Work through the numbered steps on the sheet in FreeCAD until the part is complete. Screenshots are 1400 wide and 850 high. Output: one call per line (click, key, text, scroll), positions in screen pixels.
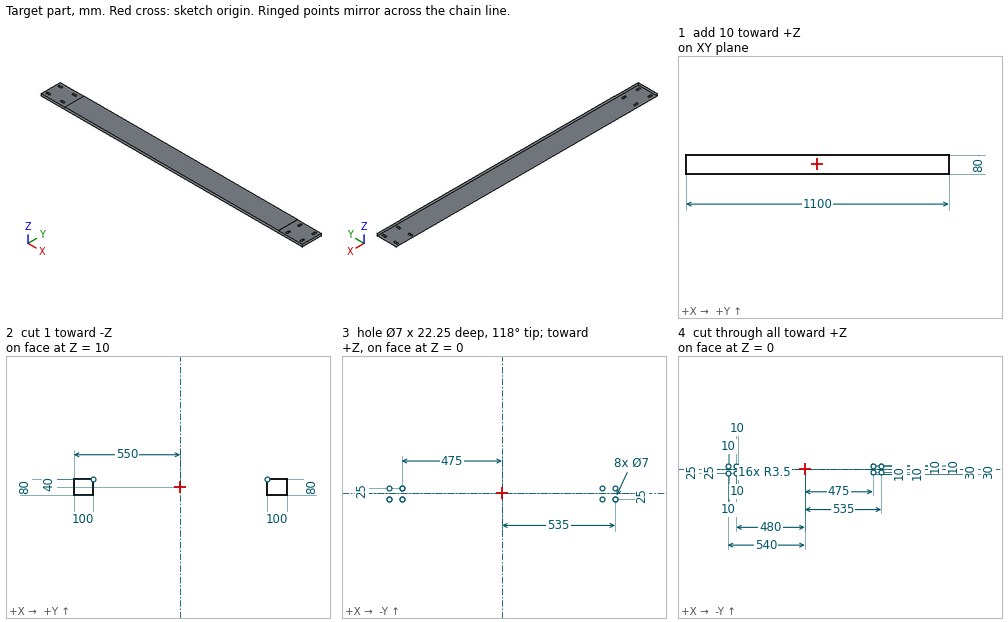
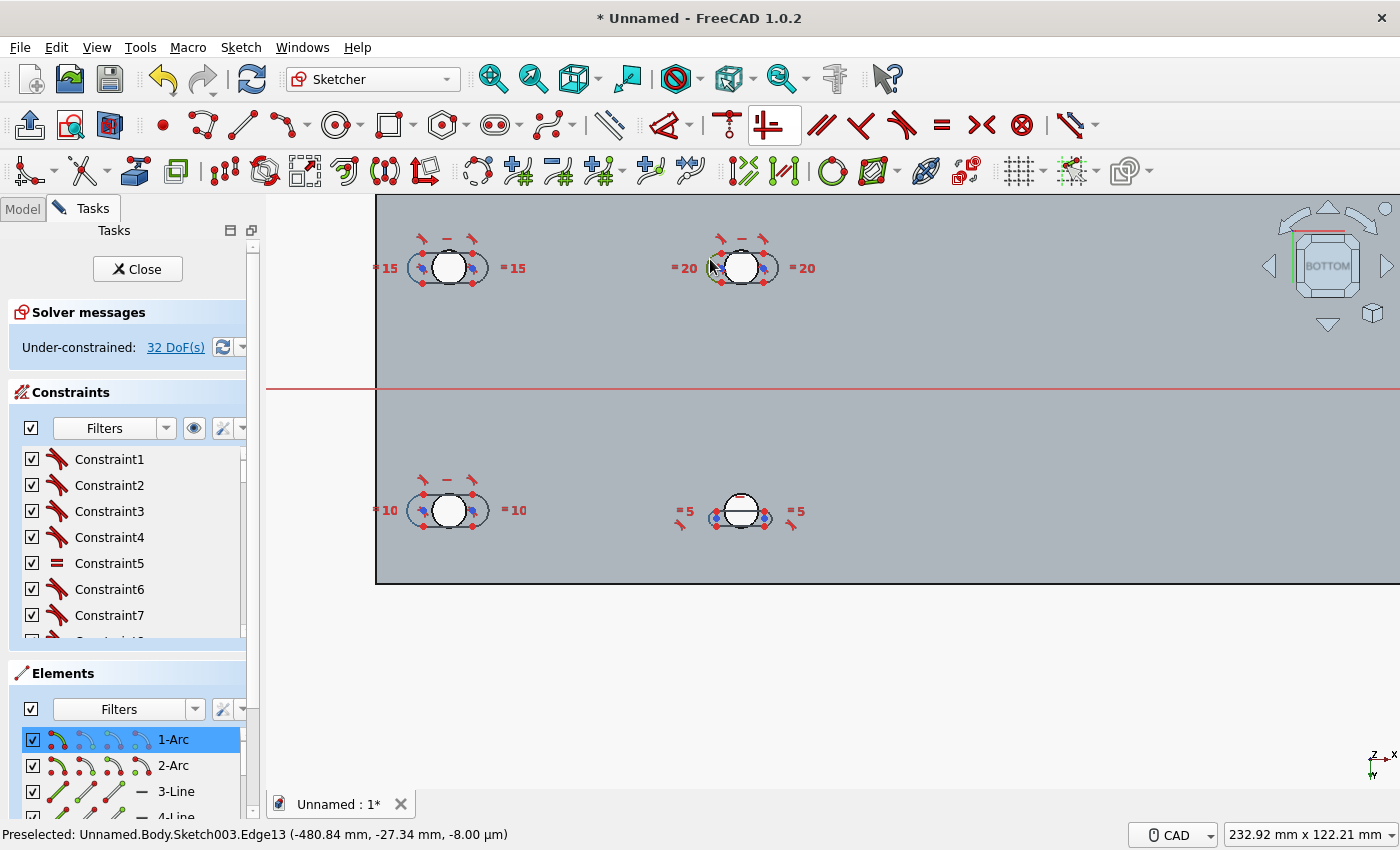
scroll(408, 508, down, 10)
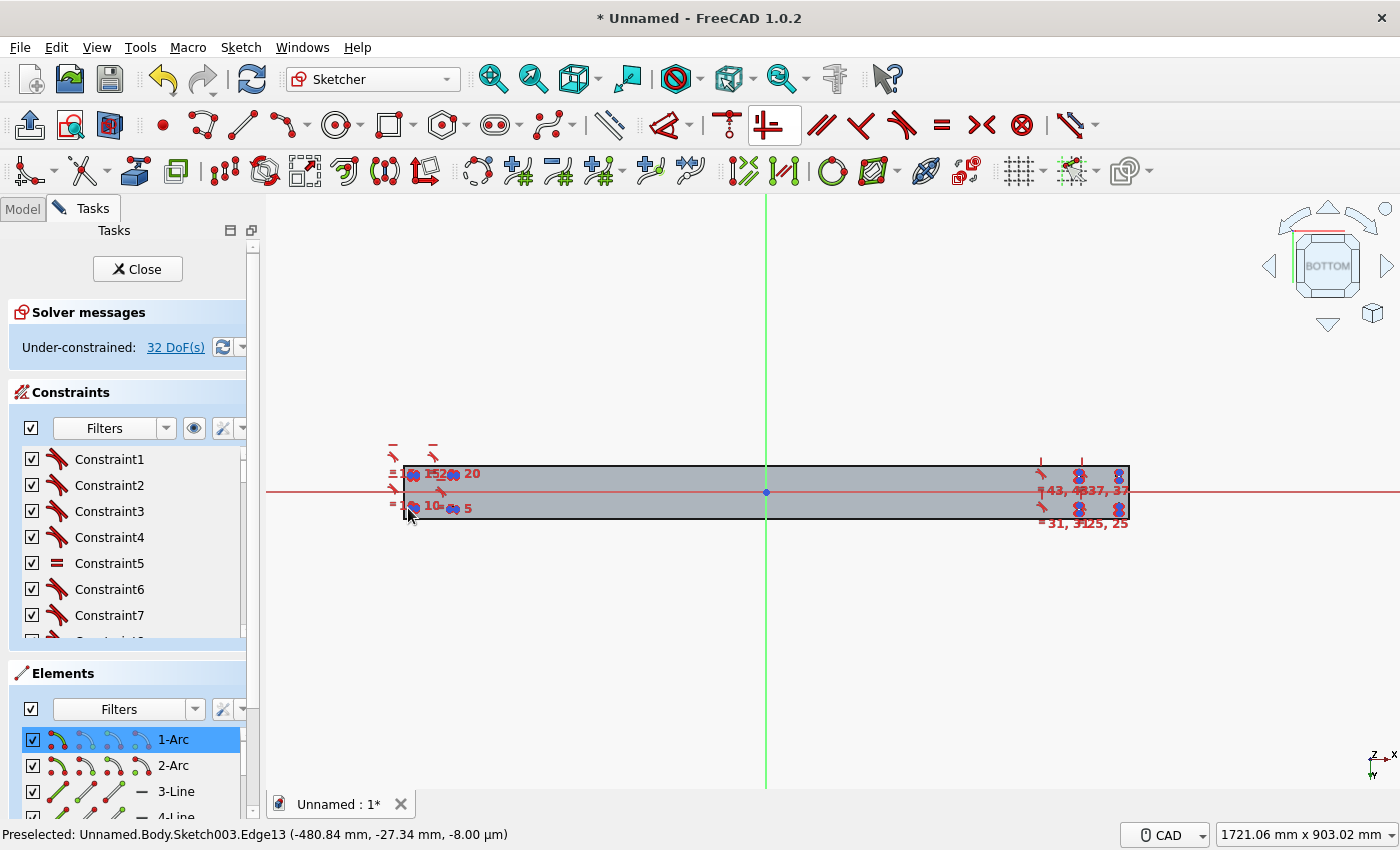
scroll(1117, 515, up, 9)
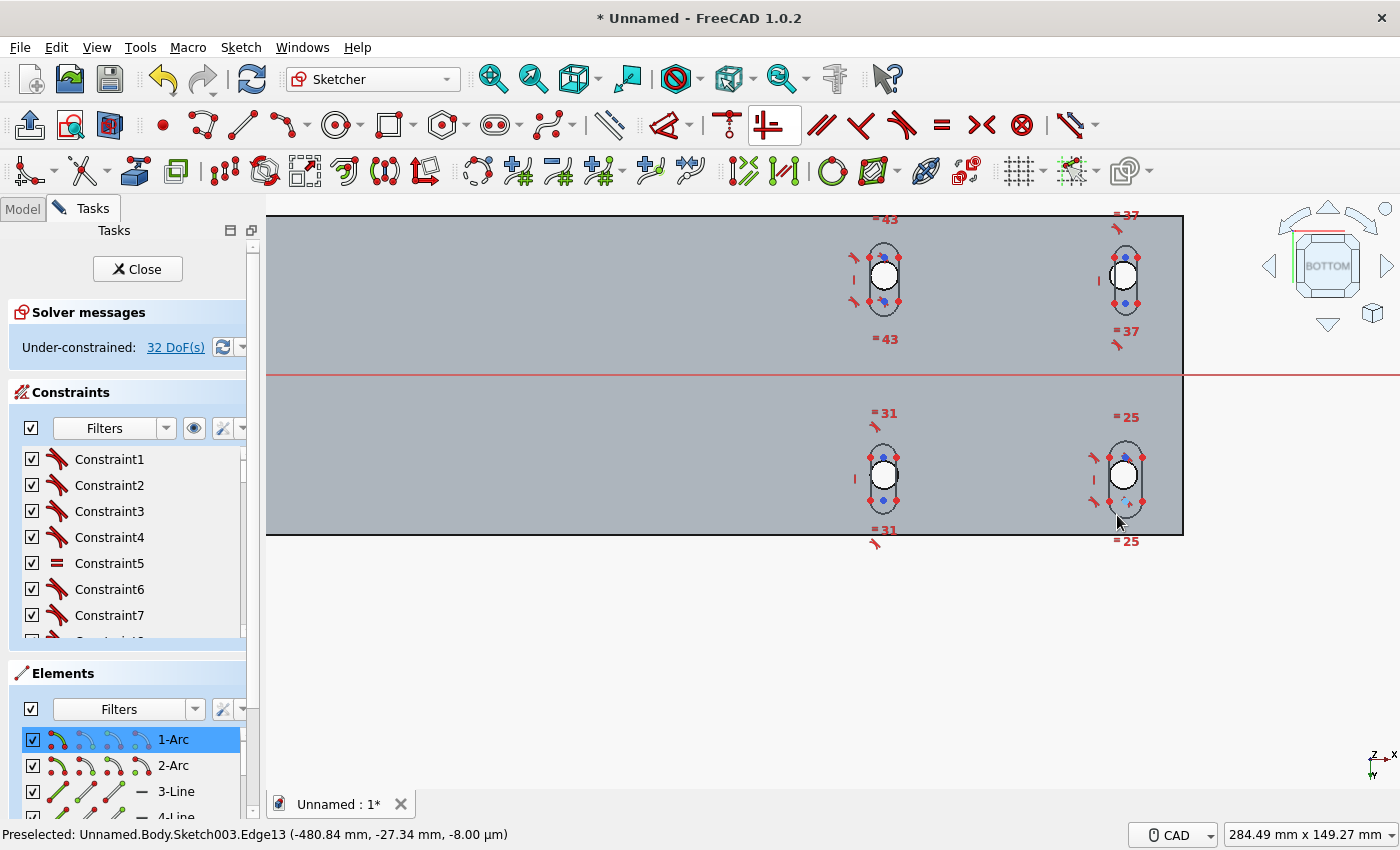
click(1116, 515)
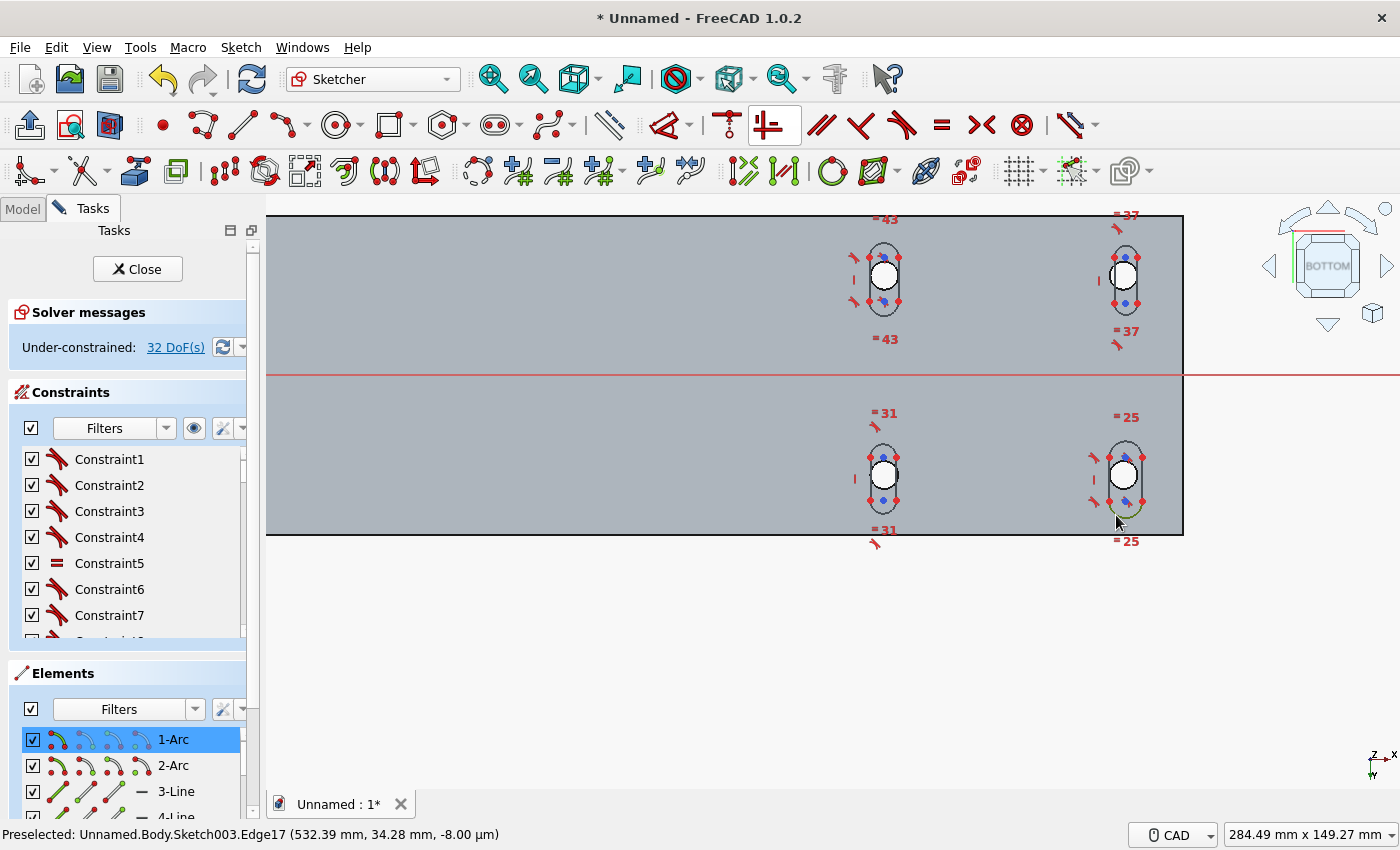
click(876, 511)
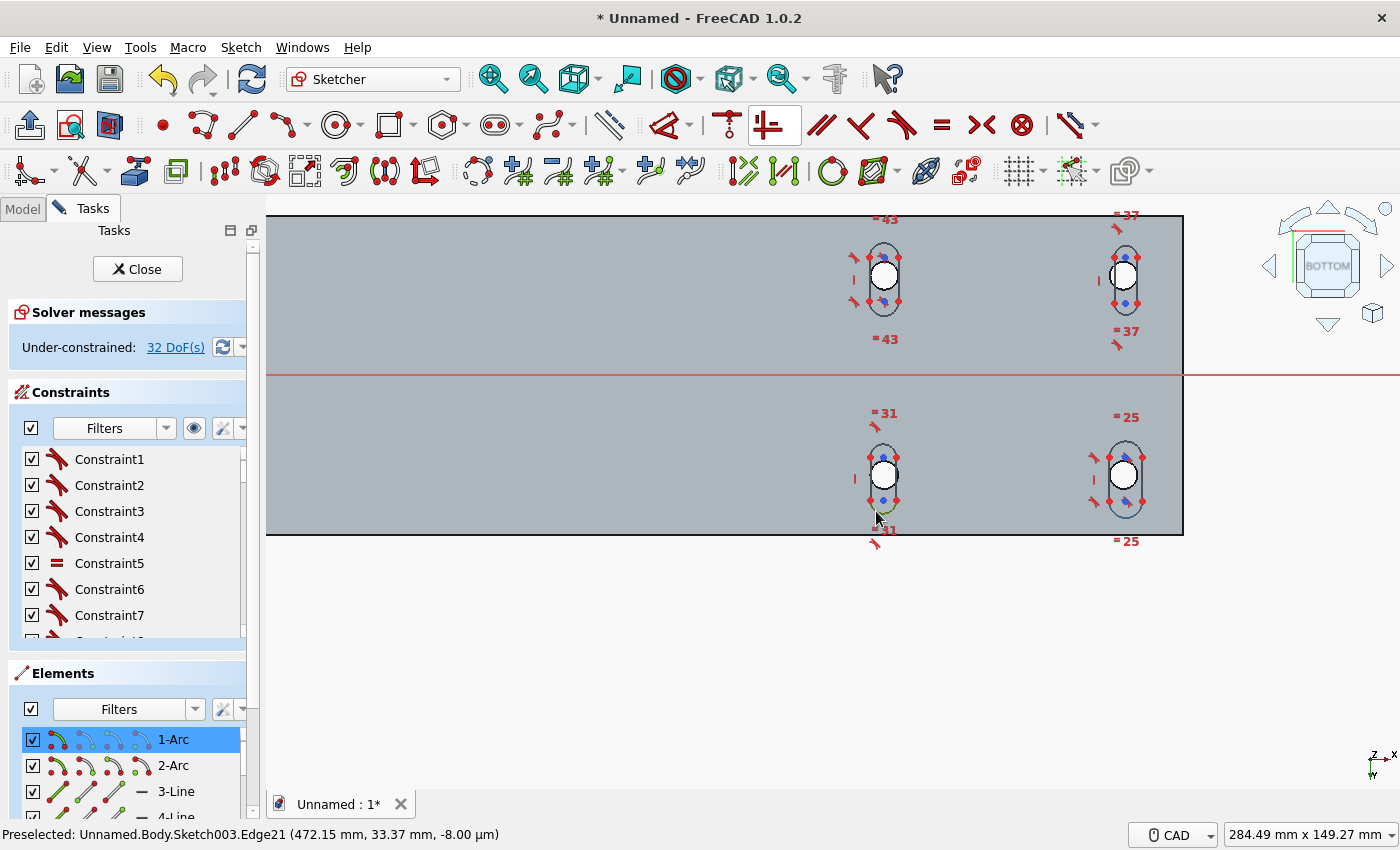
scroll(1119, 313, up, 2)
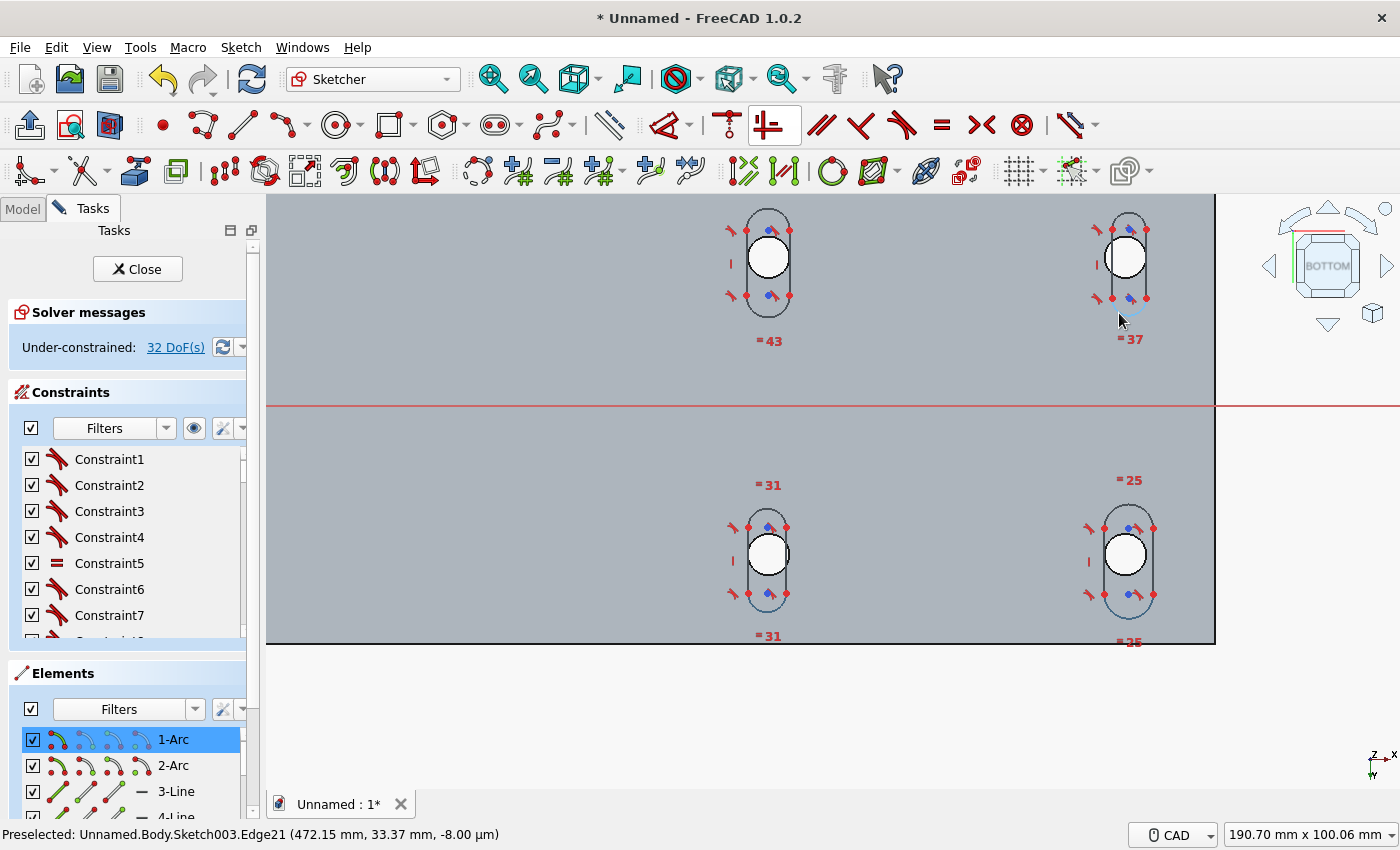
click(1119, 312)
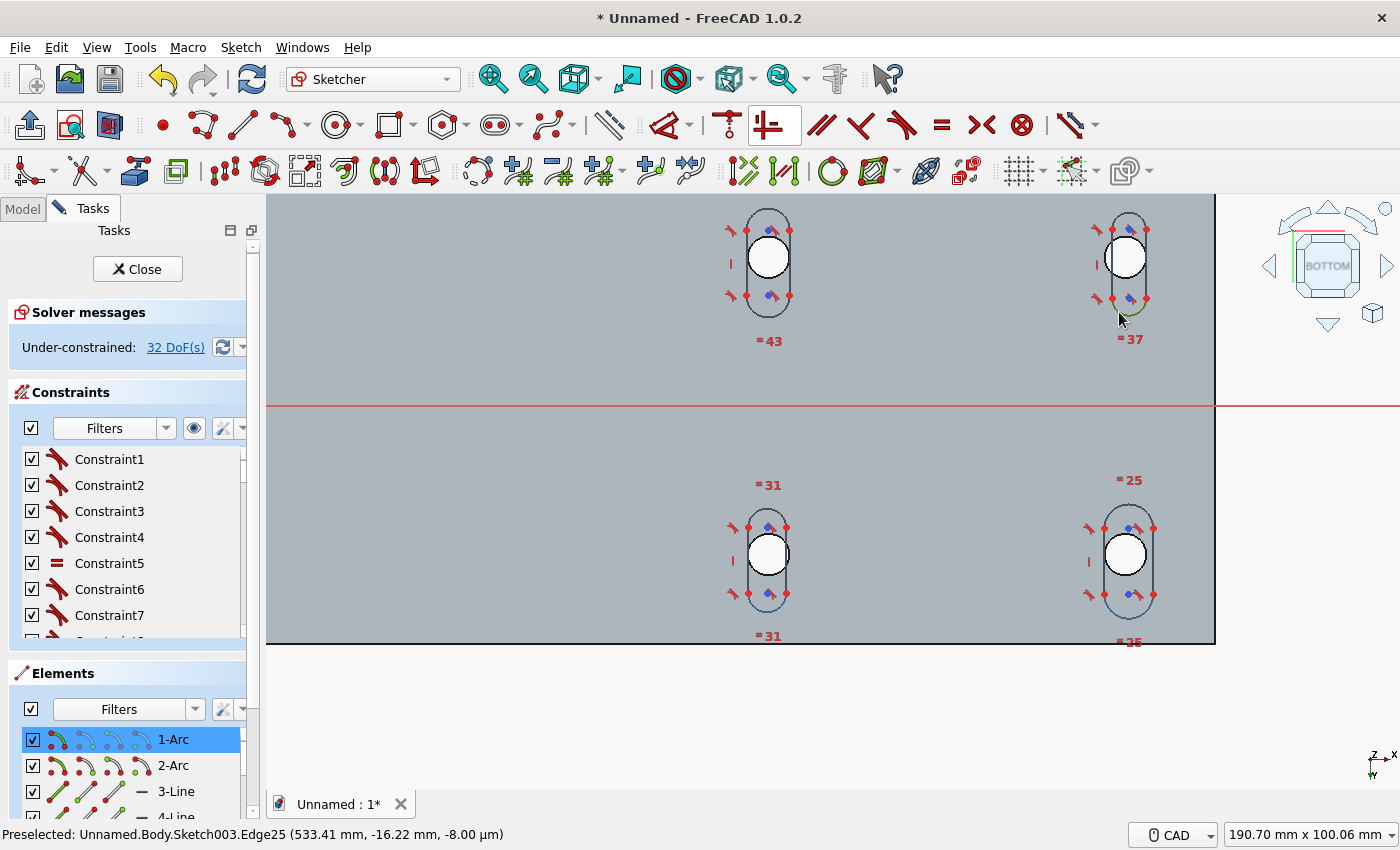
click(755, 313)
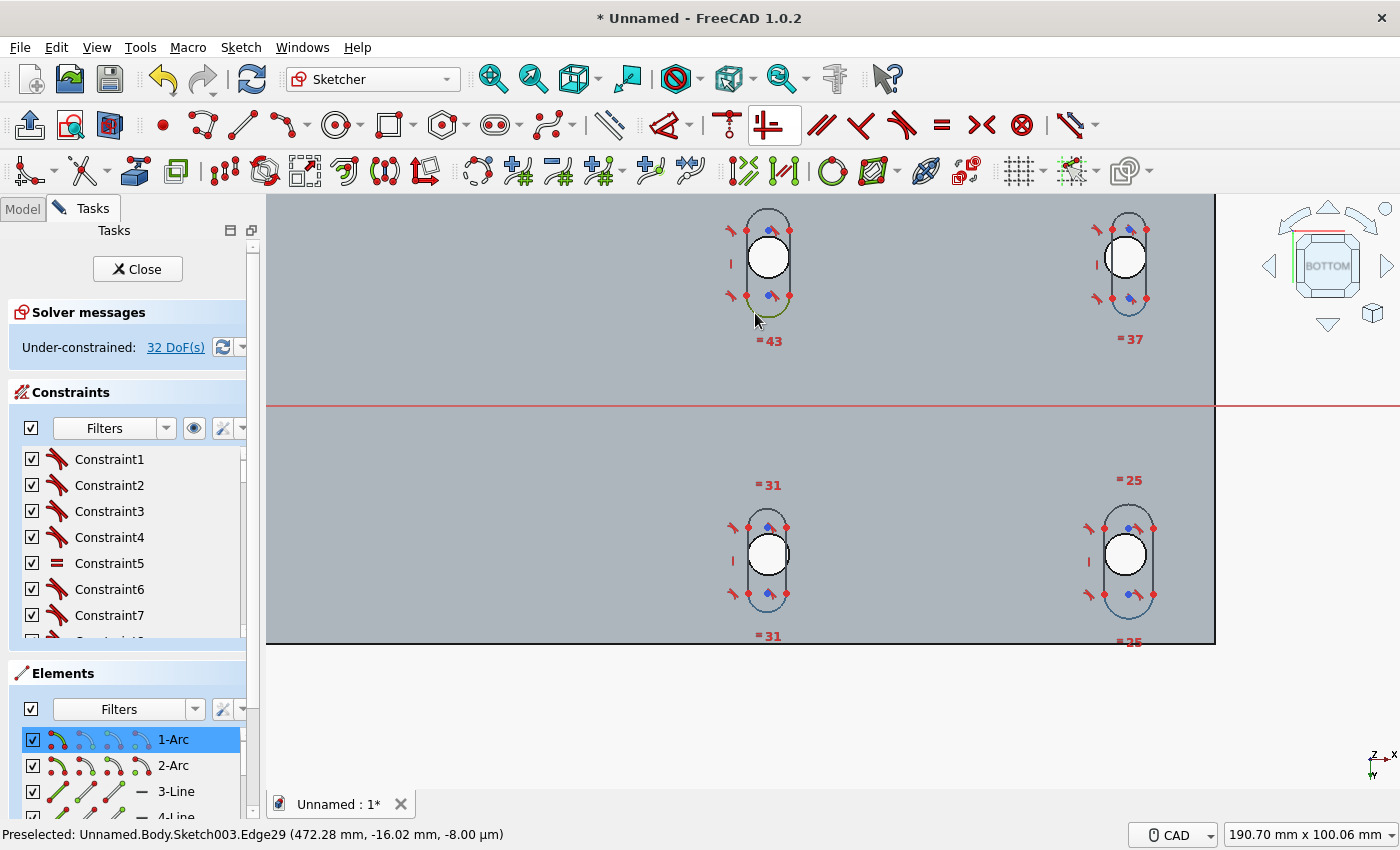
click(942, 126)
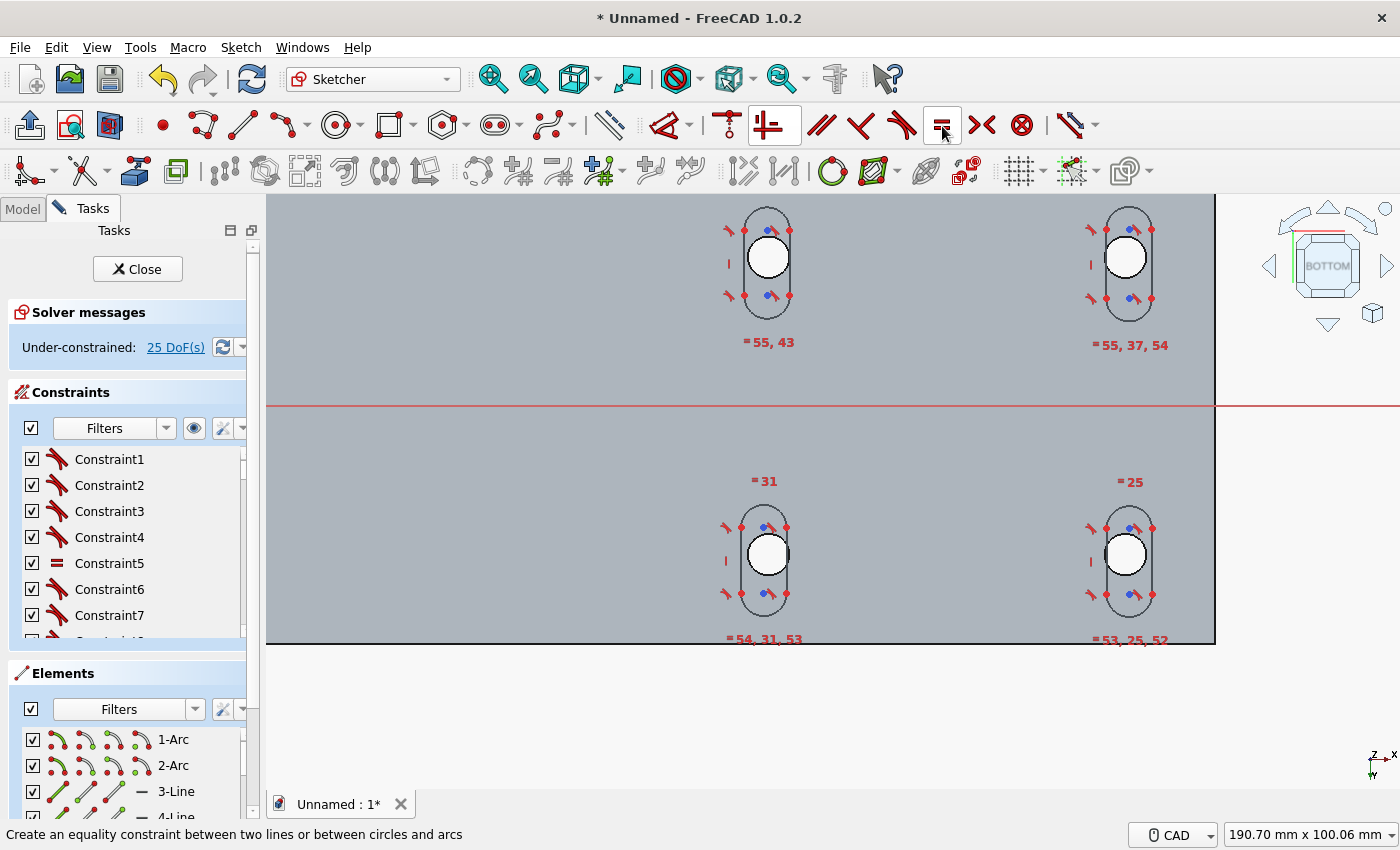
scroll(1118, 502, down, 11)